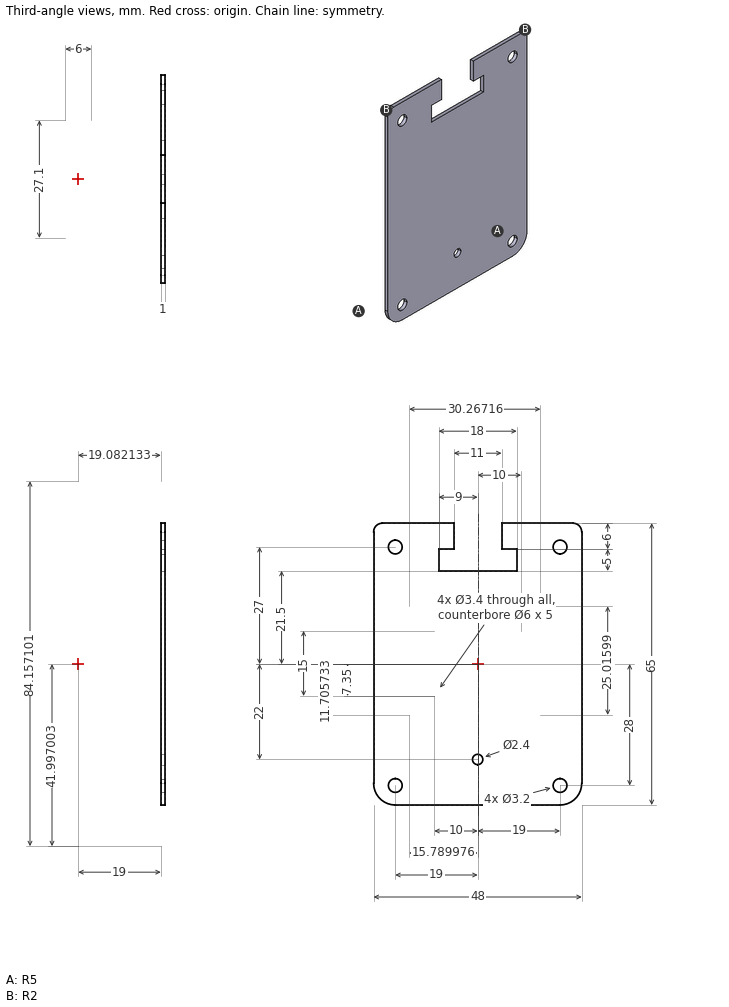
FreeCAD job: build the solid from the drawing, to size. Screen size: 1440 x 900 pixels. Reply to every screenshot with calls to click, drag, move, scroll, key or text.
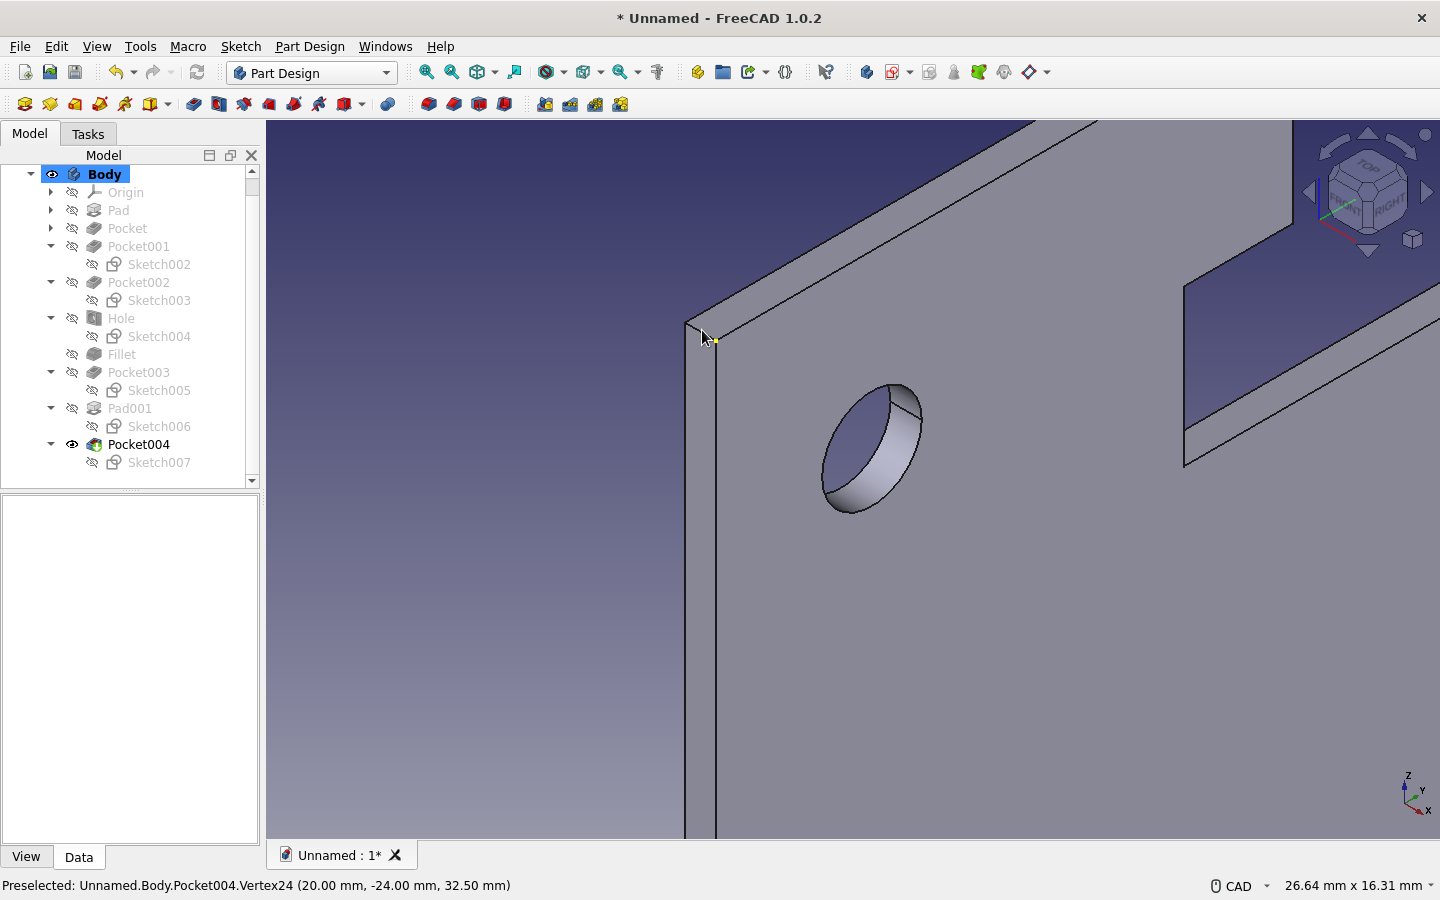
click(701, 331)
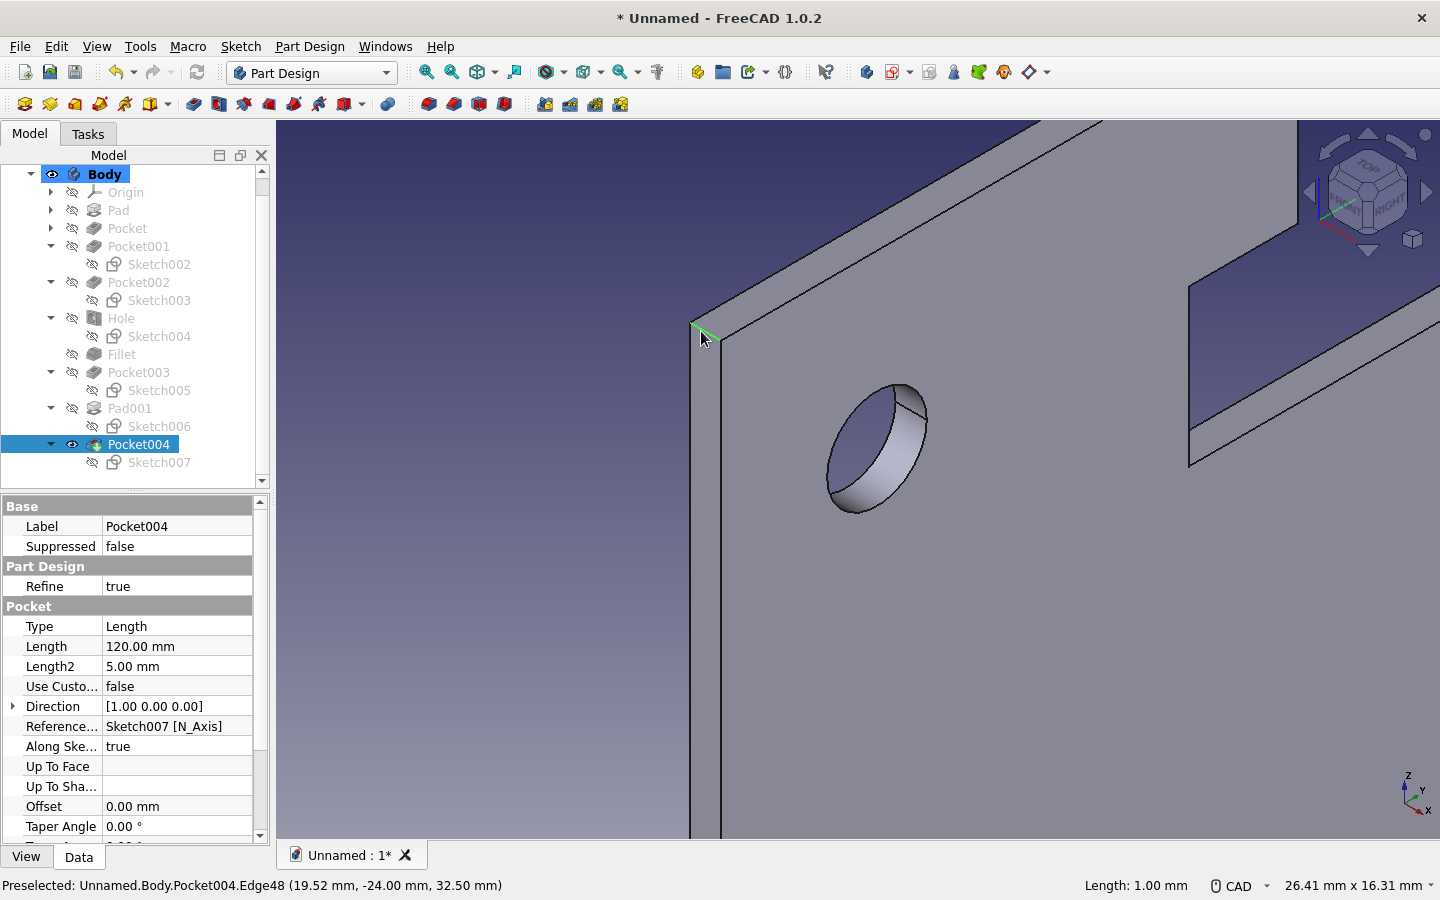
key(v)
key(f)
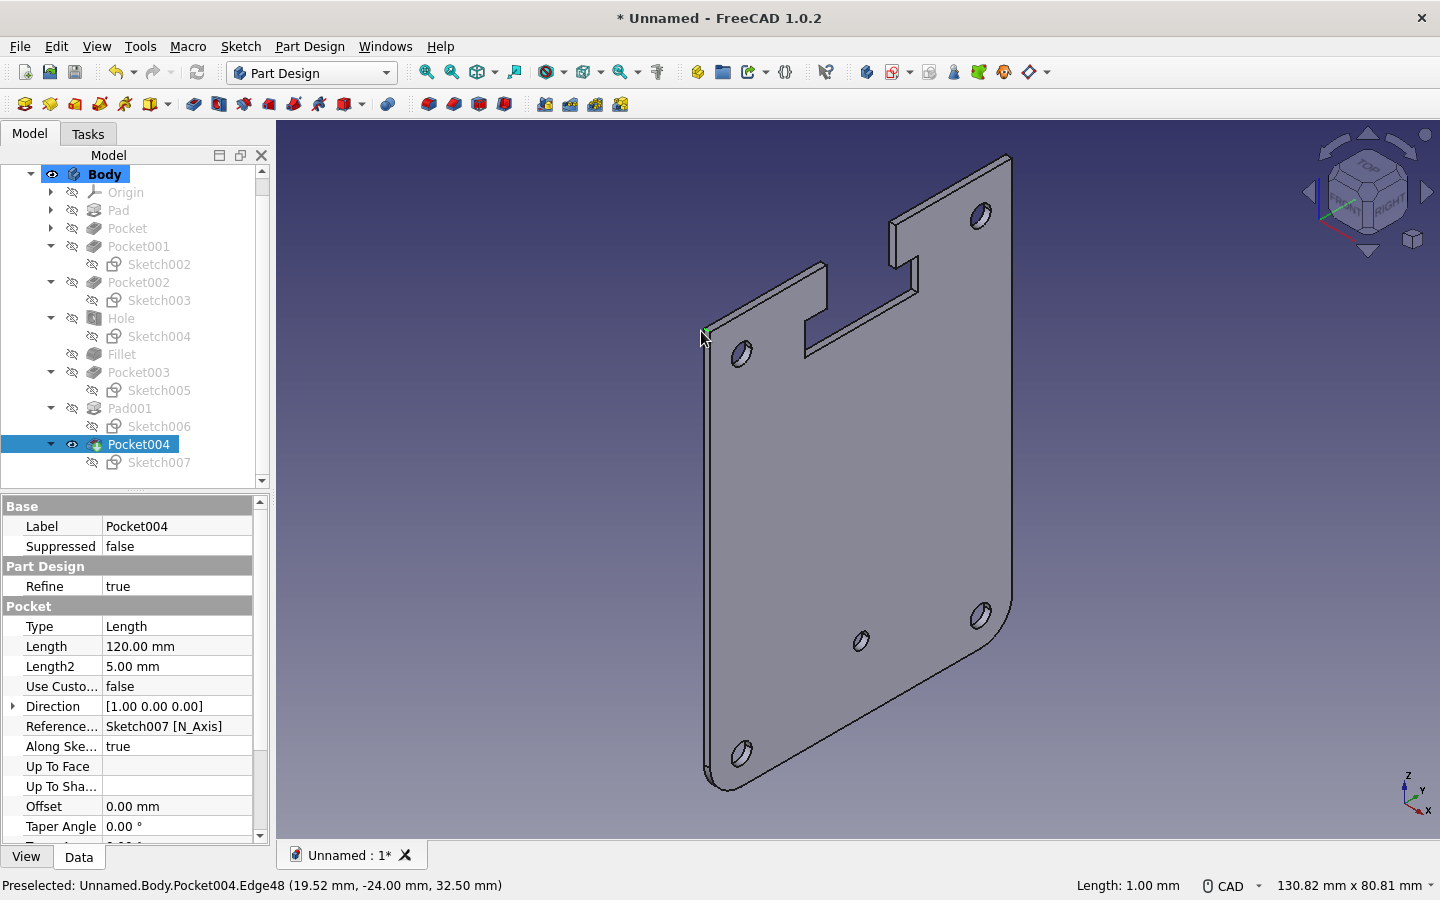
key(2)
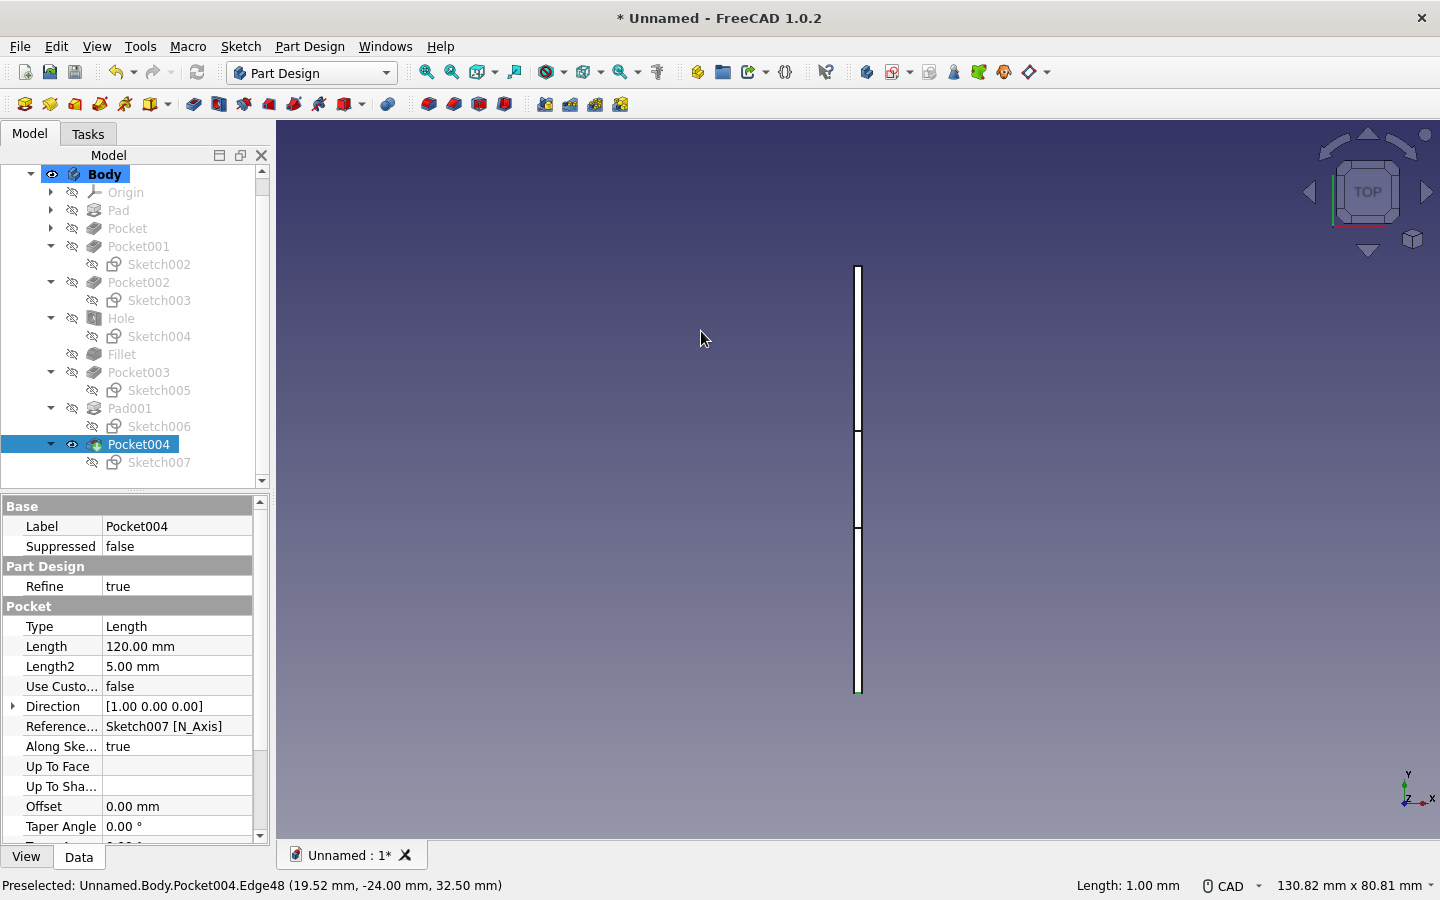
scroll(858, 265, up, 8)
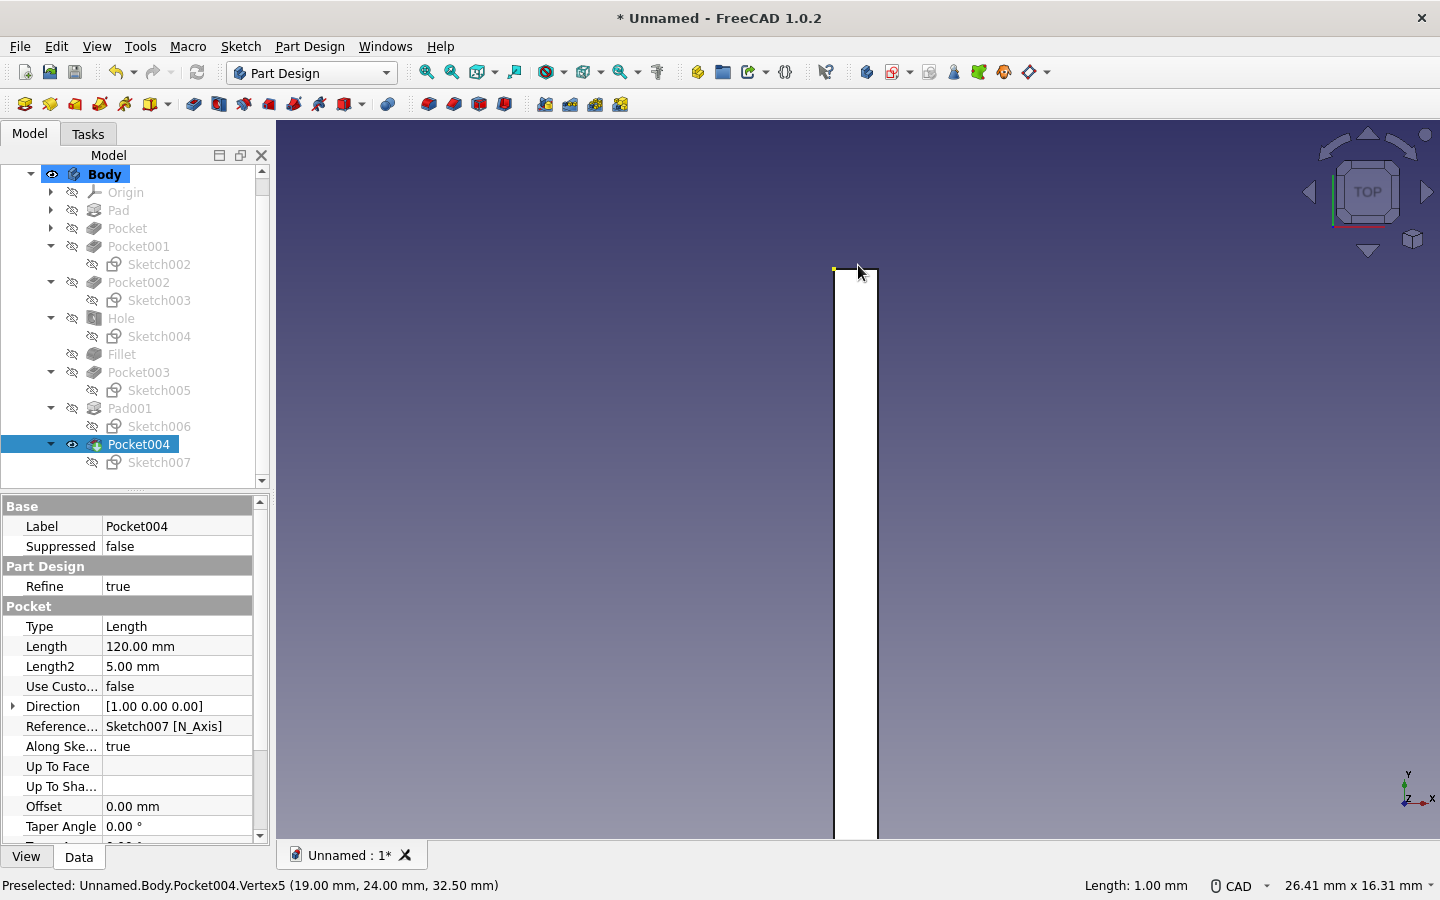
click(856, 268, ctrl)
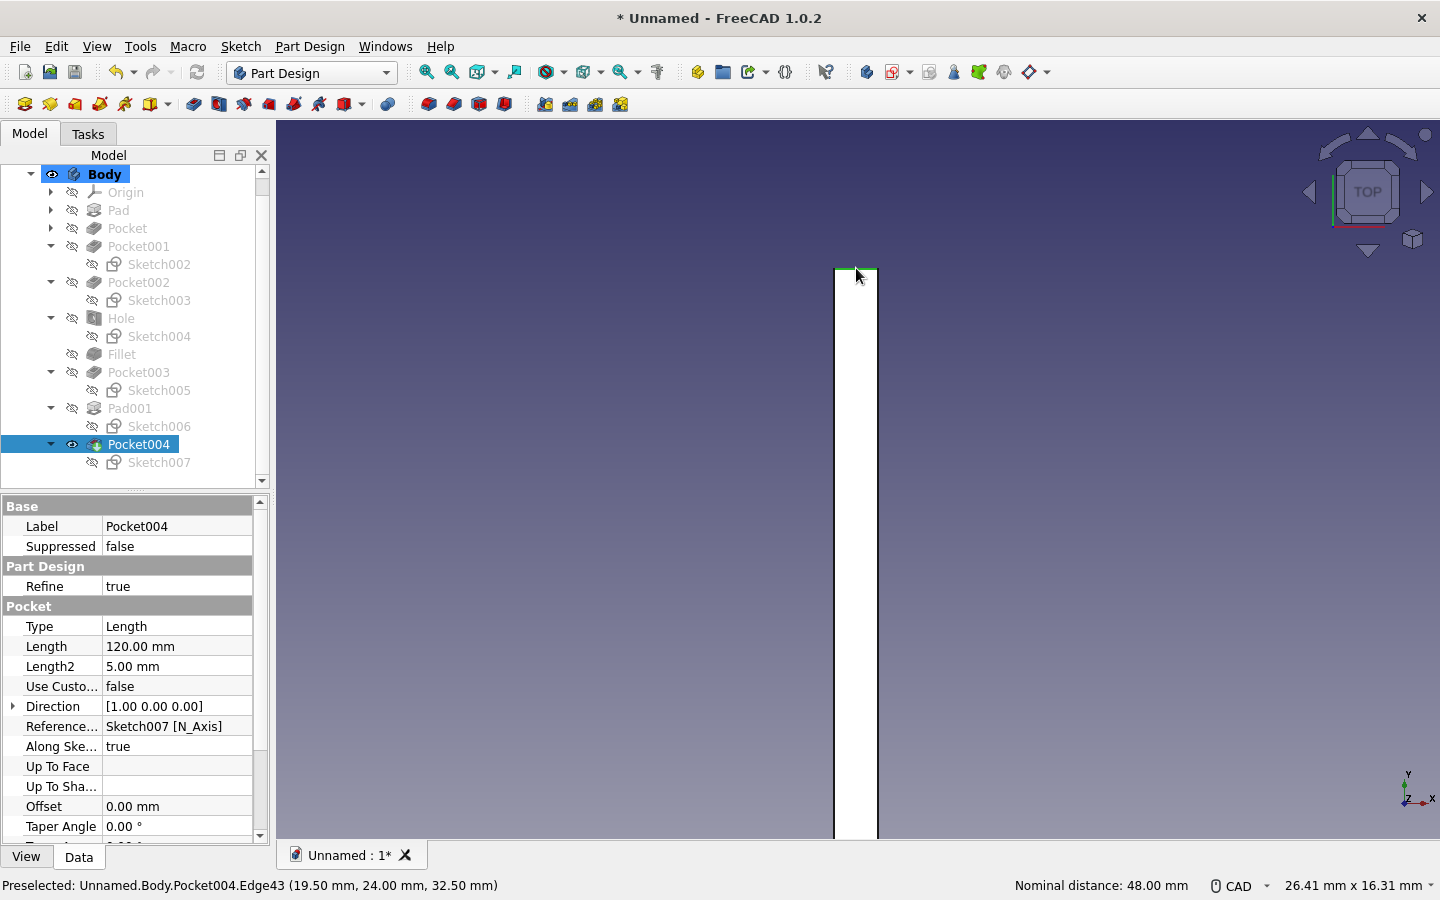
click(429, 104)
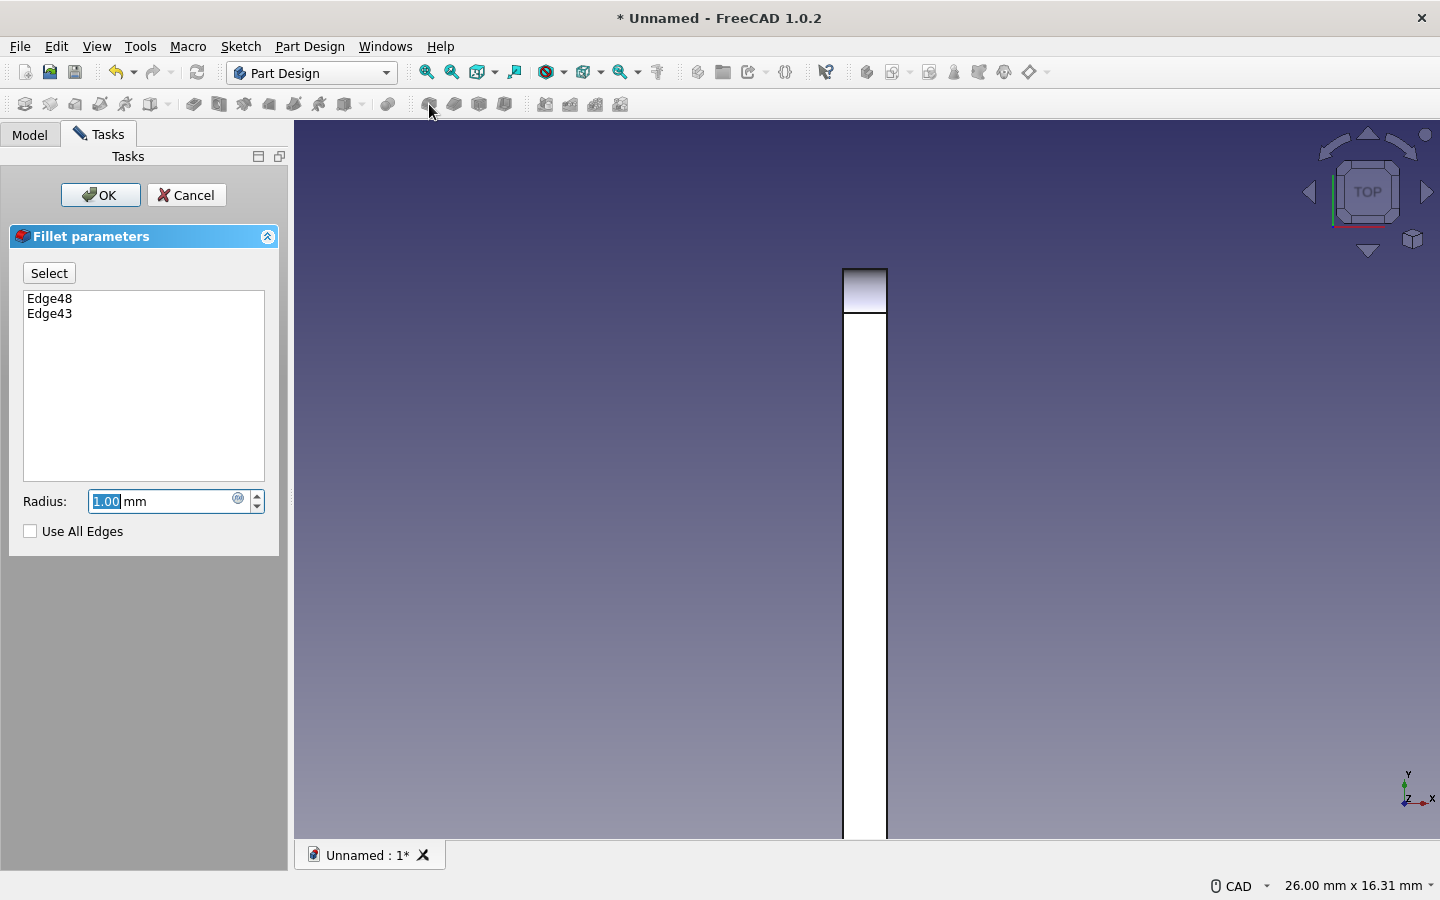
text(2)
key(Tab)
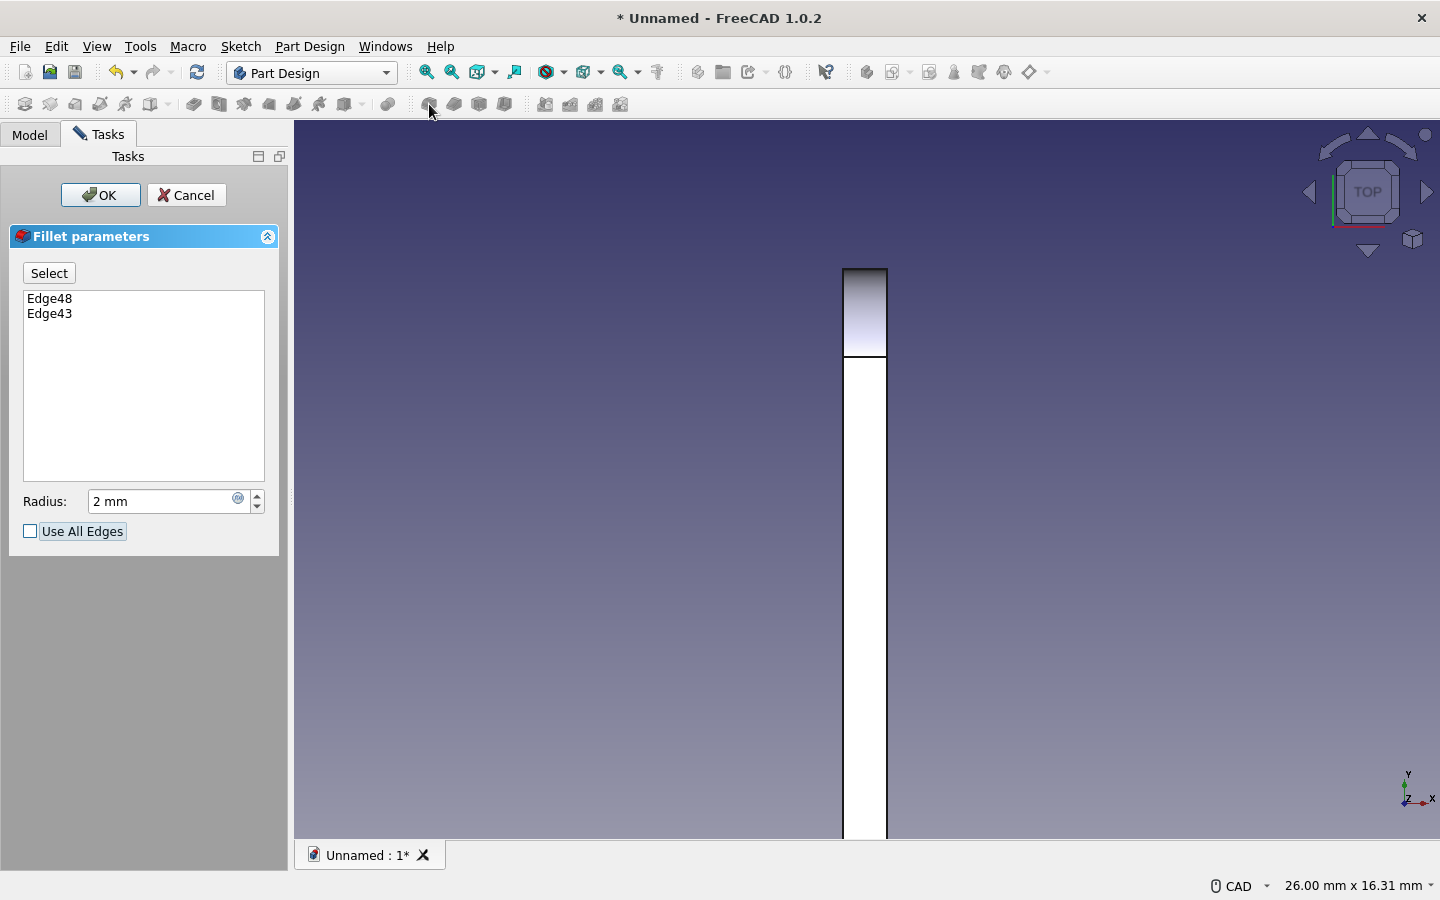
click(101, 195)